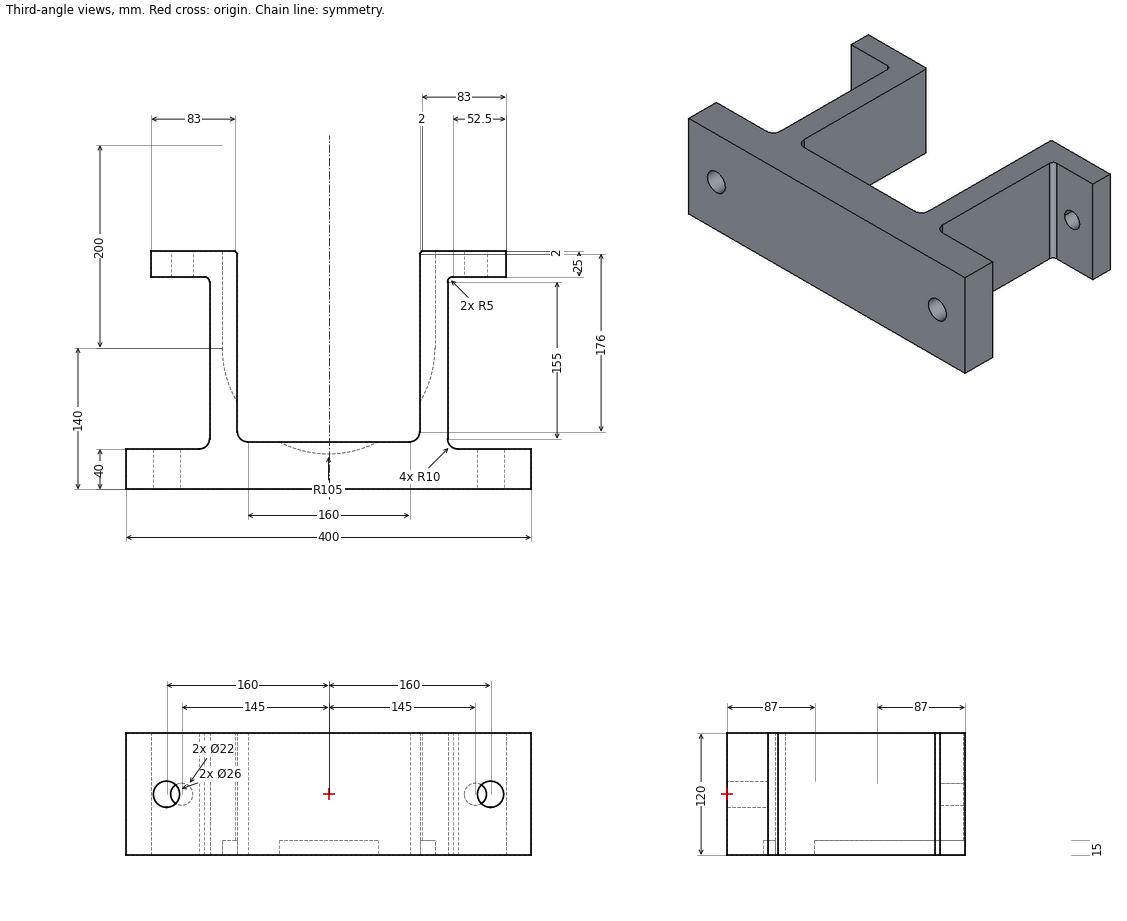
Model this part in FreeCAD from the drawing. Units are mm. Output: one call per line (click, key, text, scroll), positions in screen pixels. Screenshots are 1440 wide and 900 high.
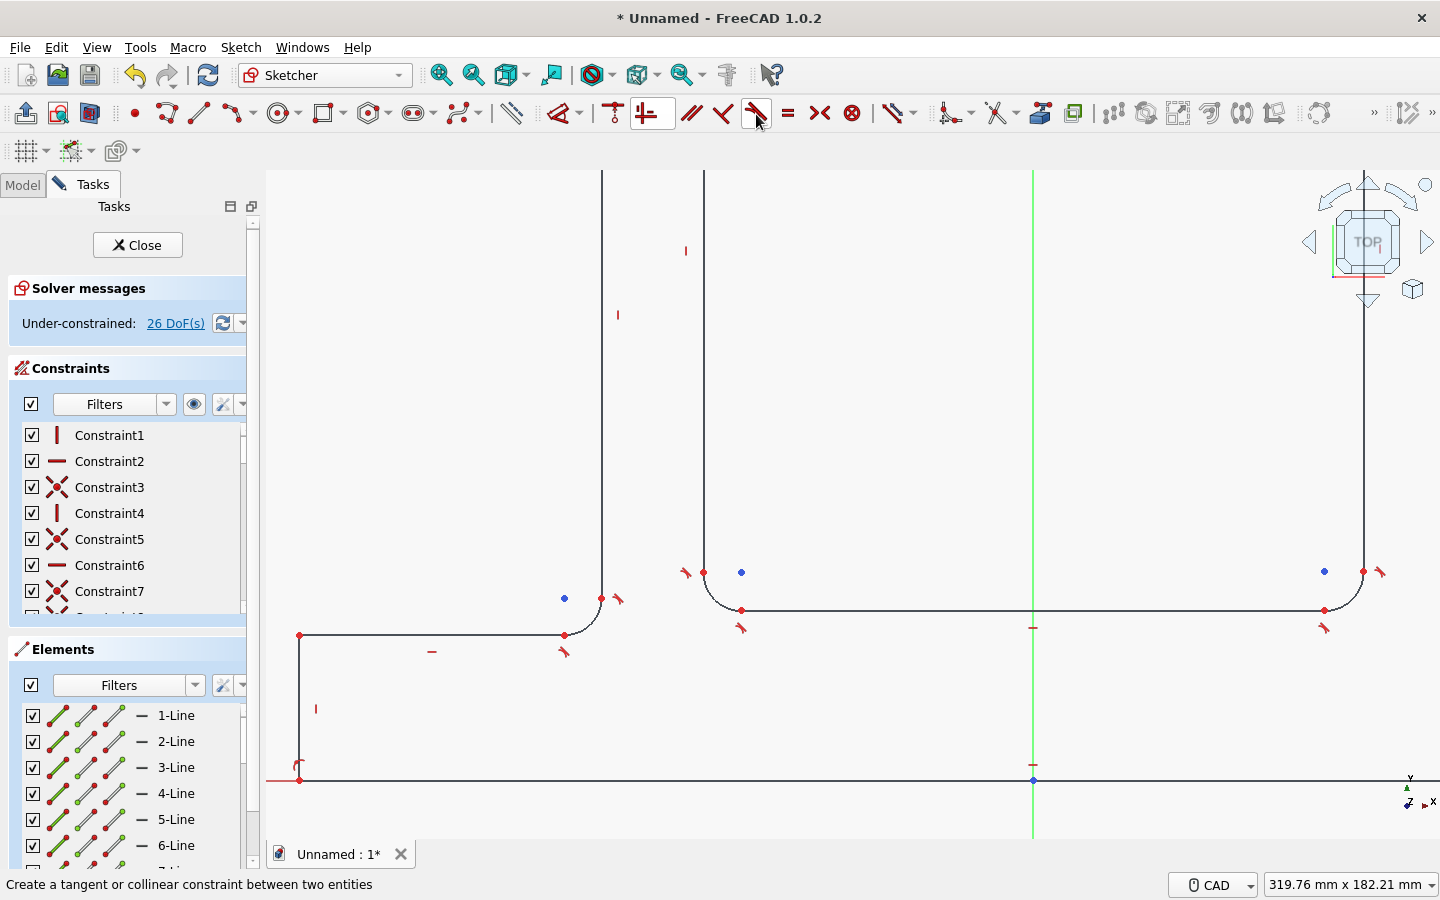
scroll(582, 631, down, 4)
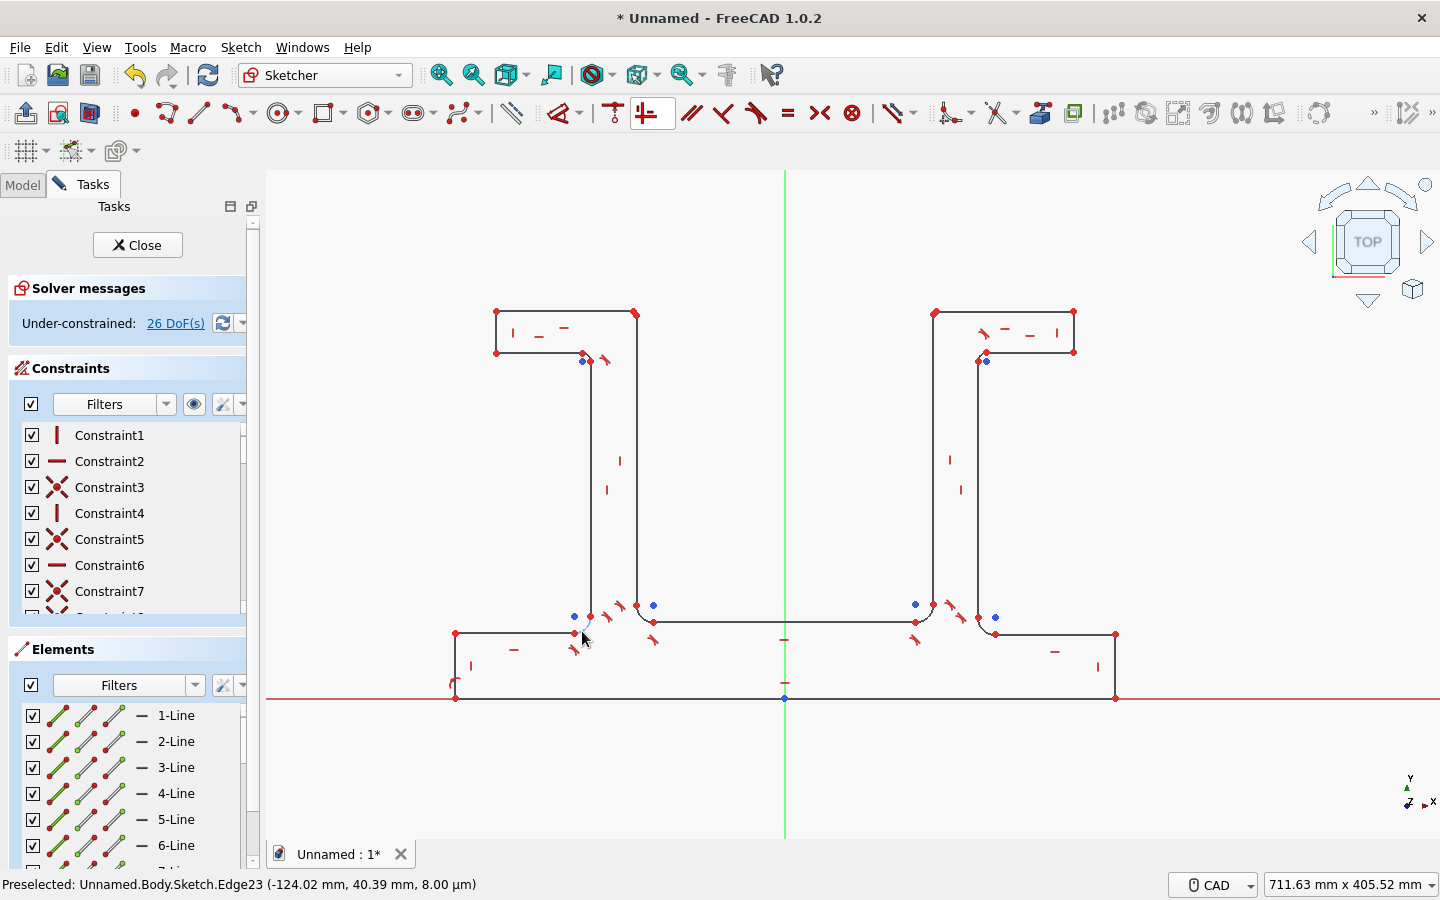
click(1079, 635)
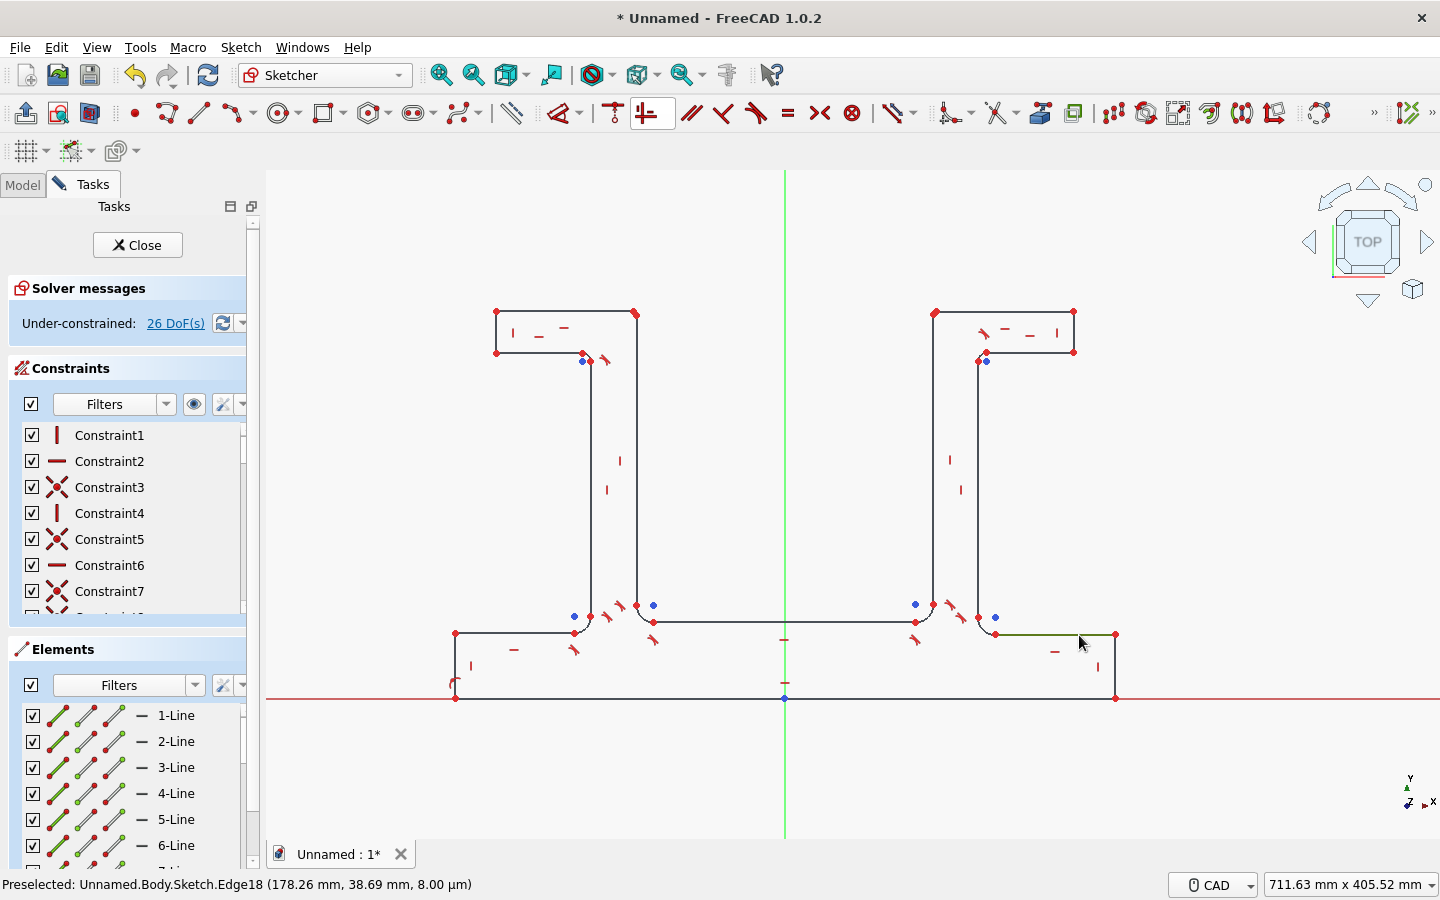
click(983, 630)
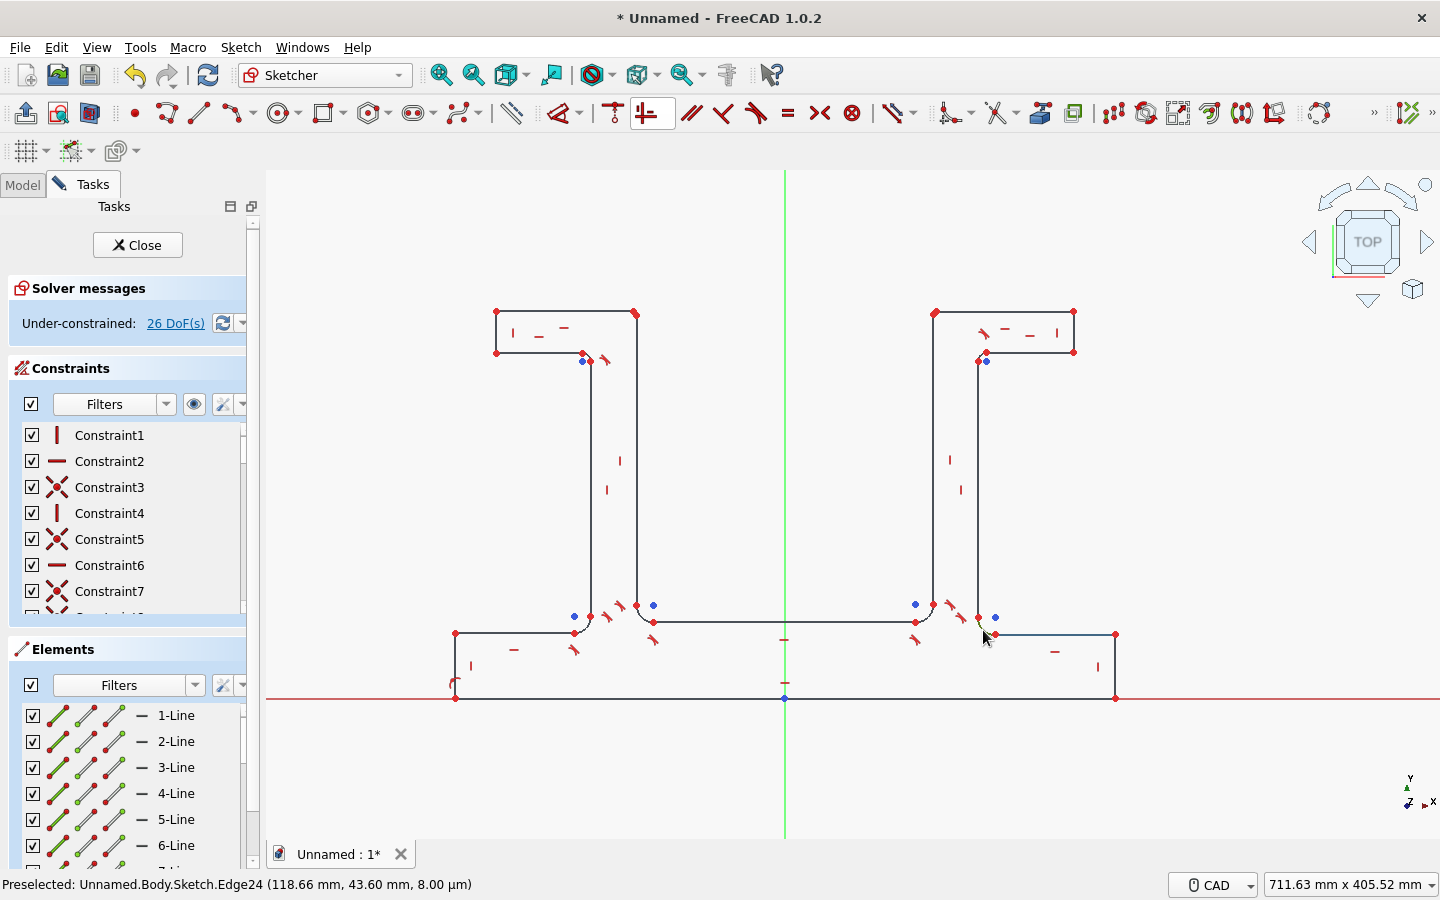
click(756, 114)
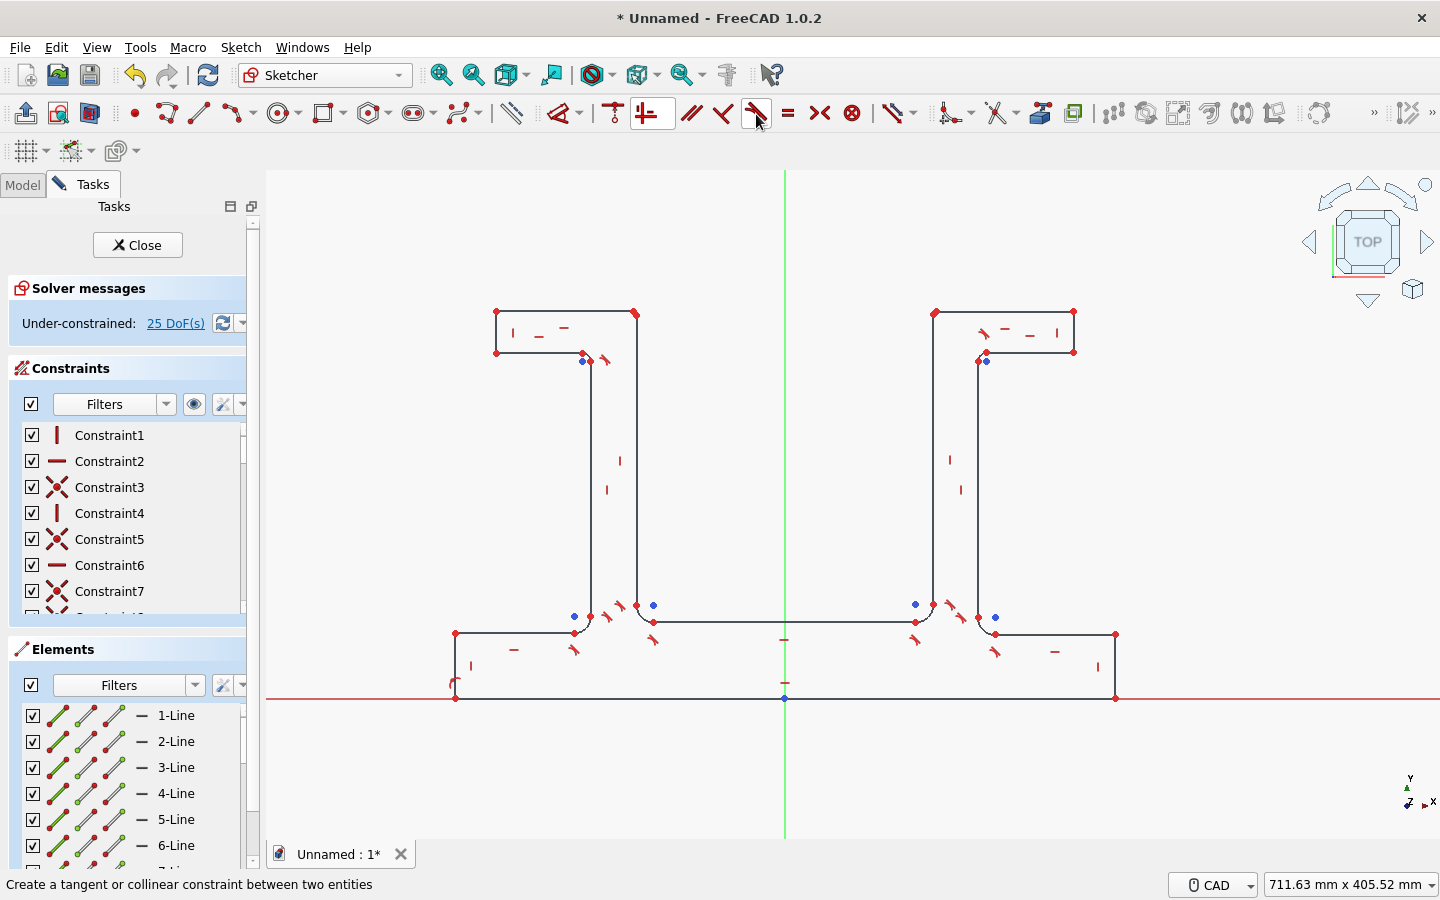
click(928, 617)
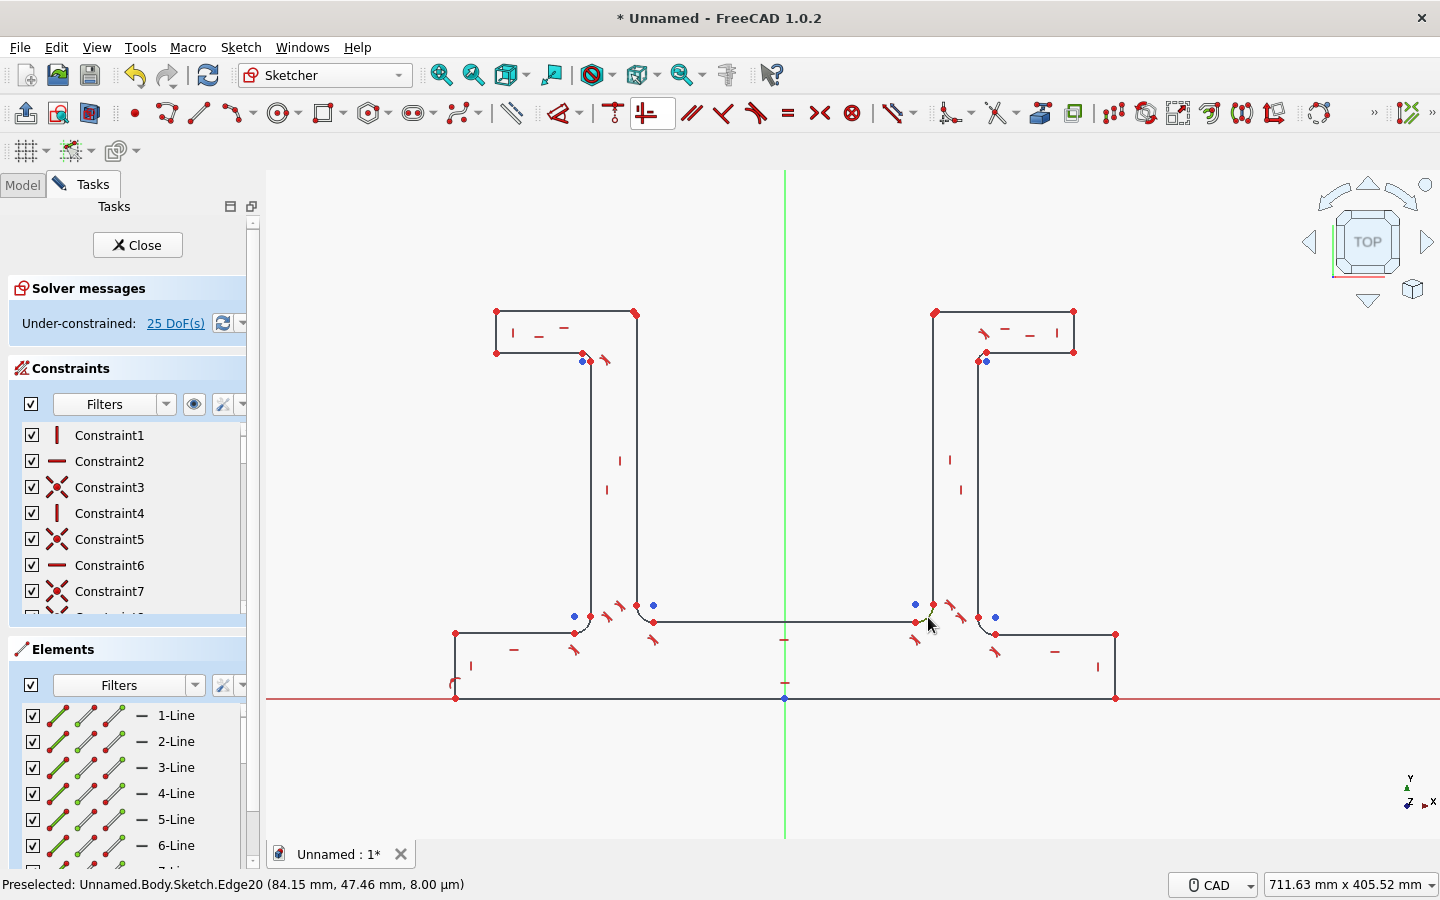
click(642, 617)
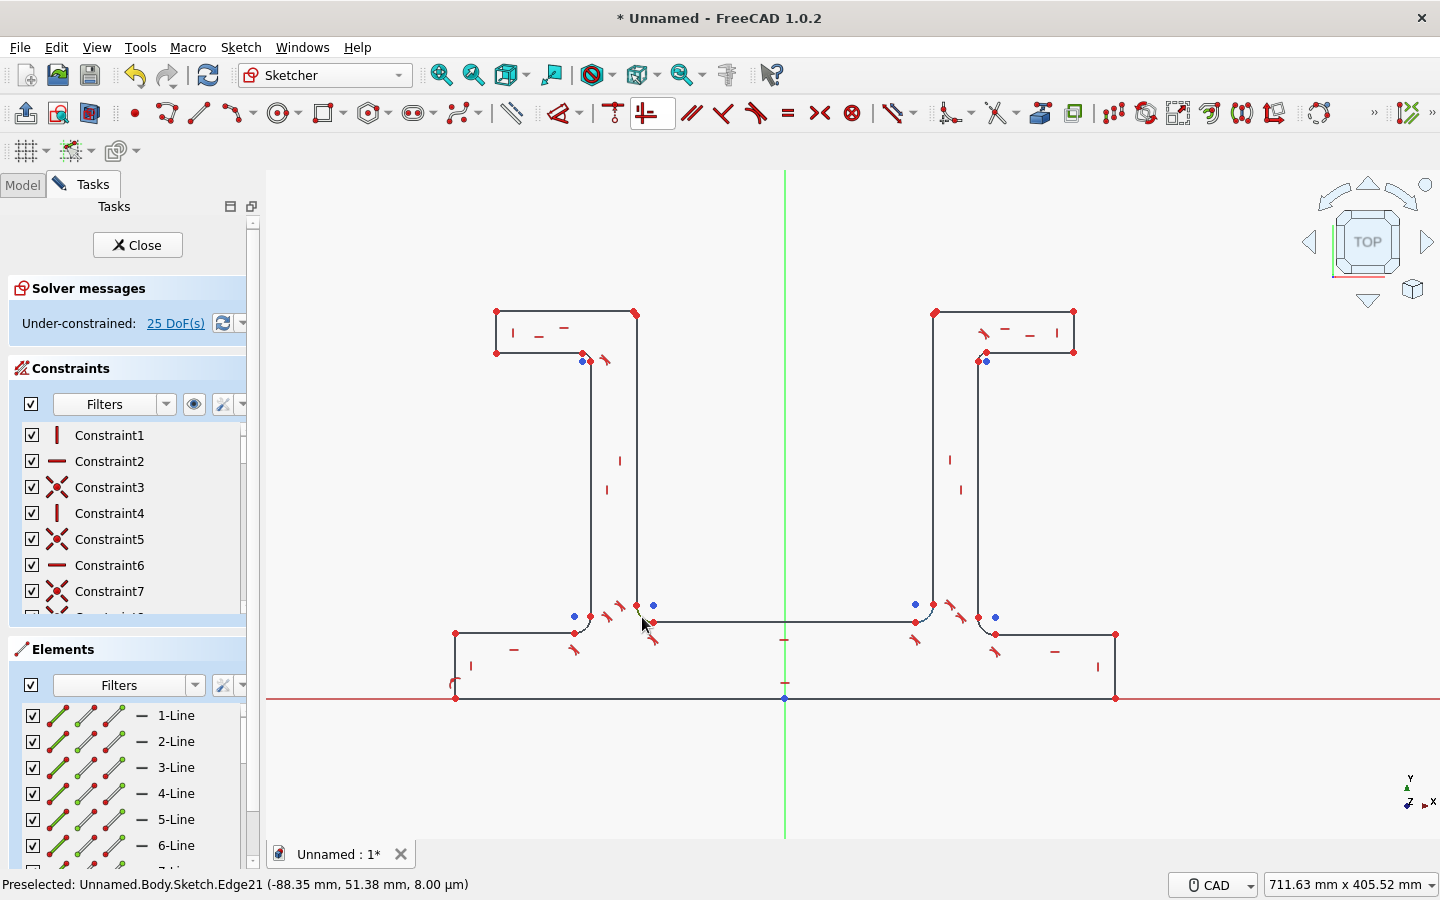
click(586, 628)